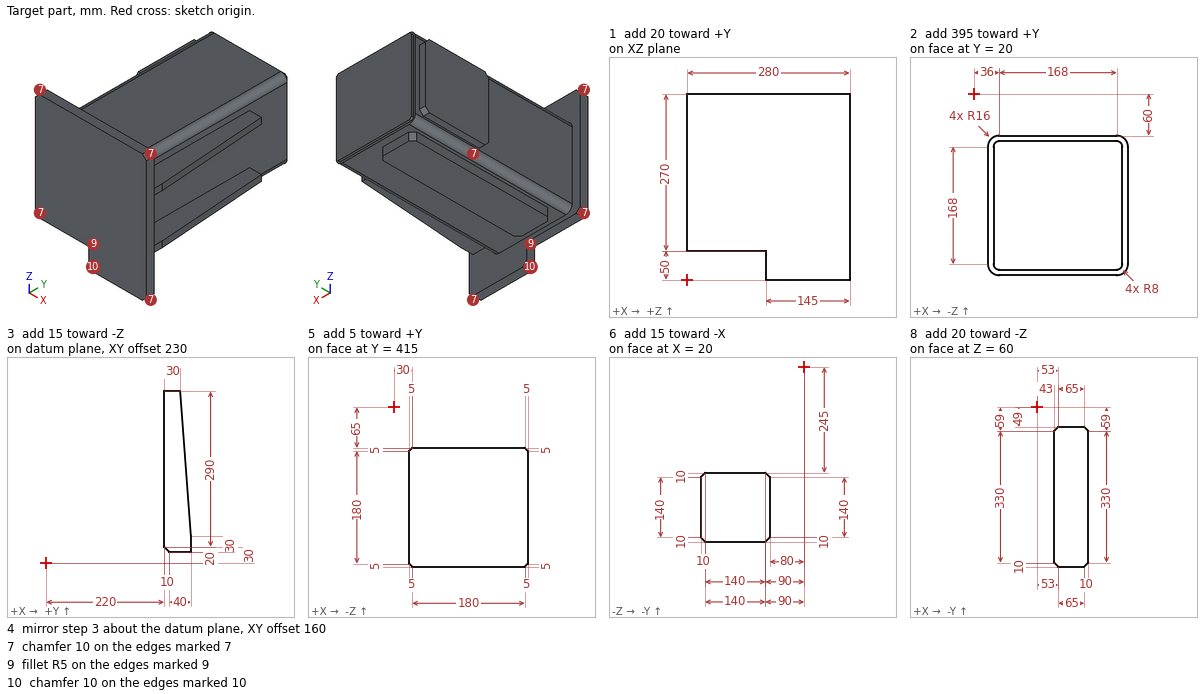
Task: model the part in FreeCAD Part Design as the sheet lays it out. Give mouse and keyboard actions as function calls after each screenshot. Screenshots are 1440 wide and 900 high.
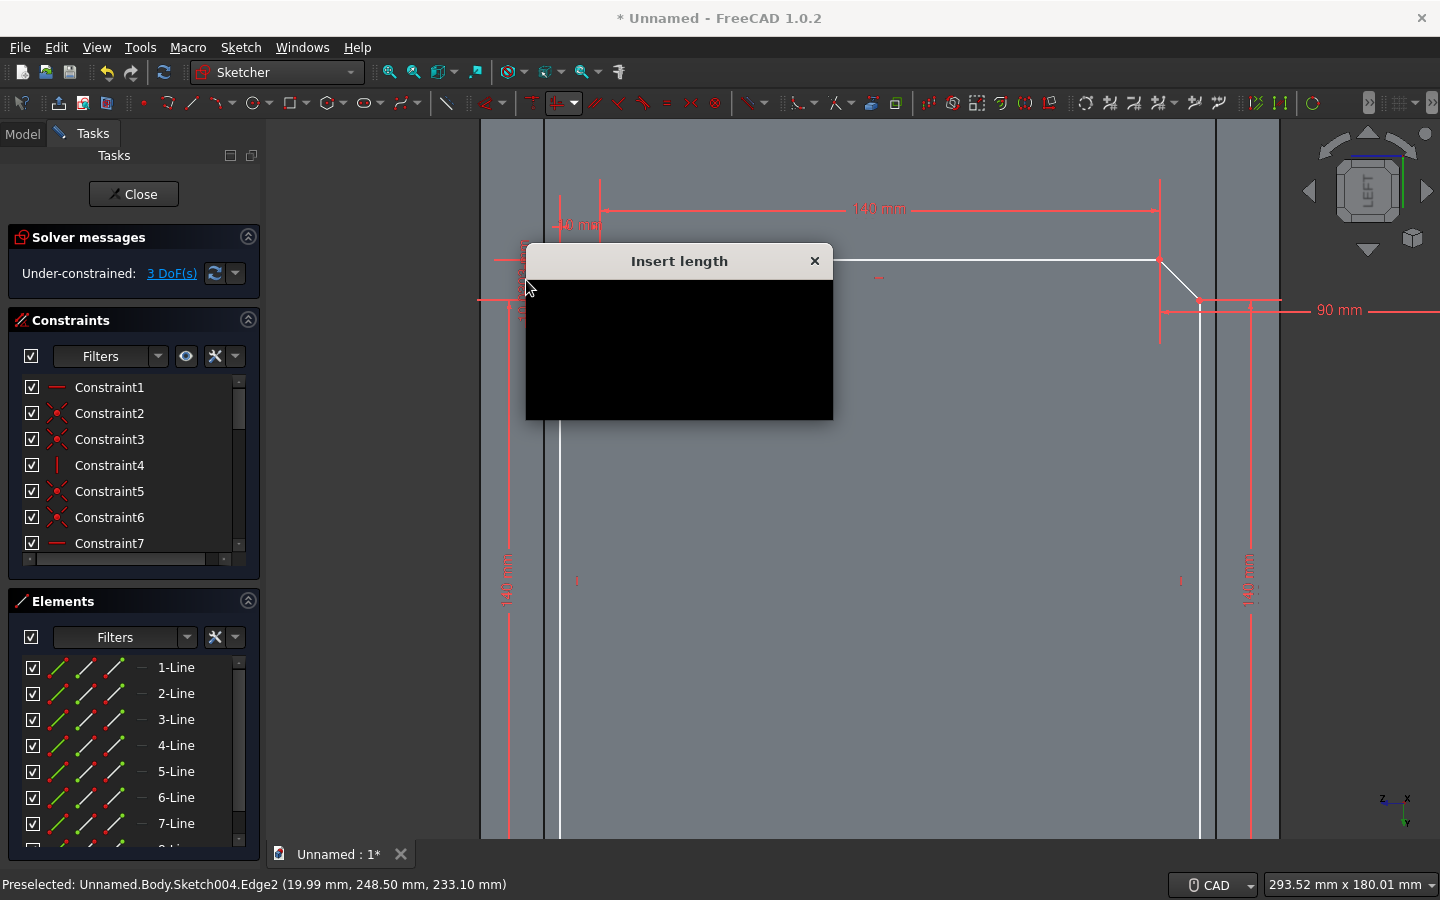
text(10)
key(Return)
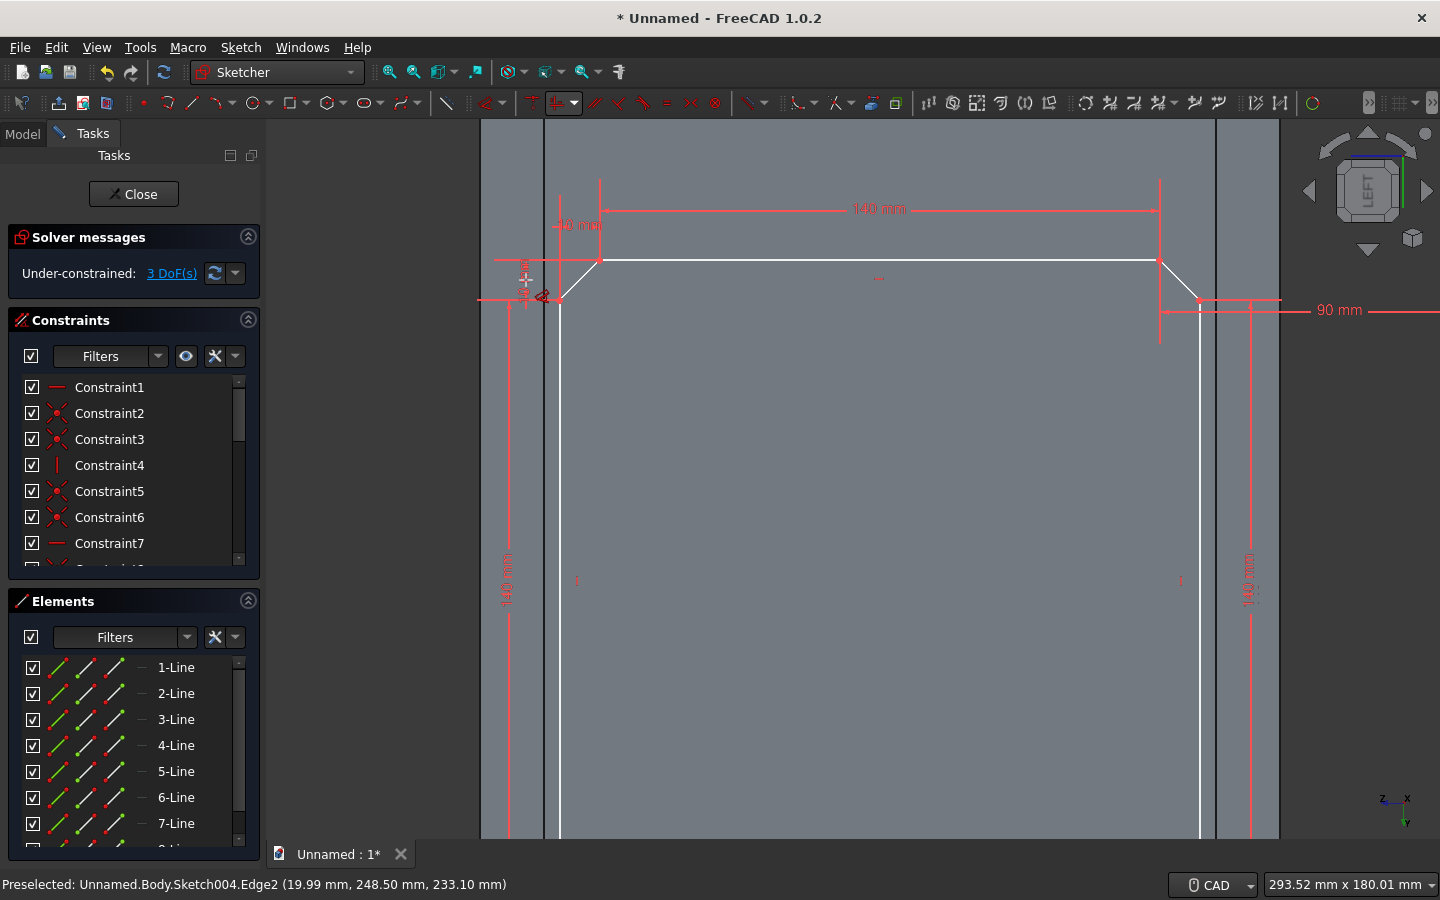
scroll(591, 277, down, 2)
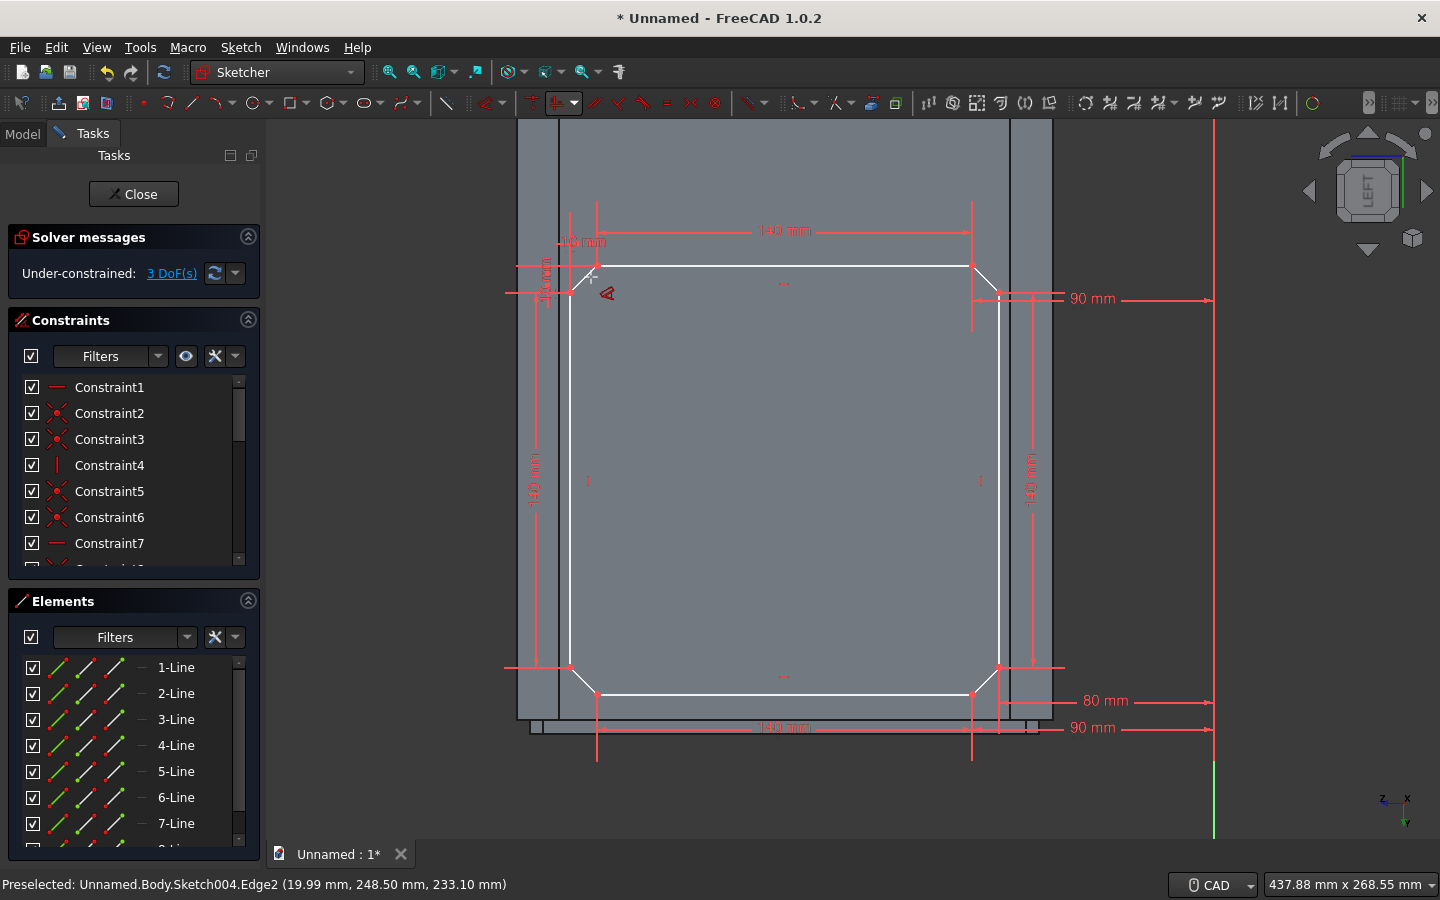
scroll(578, 676, up, 2)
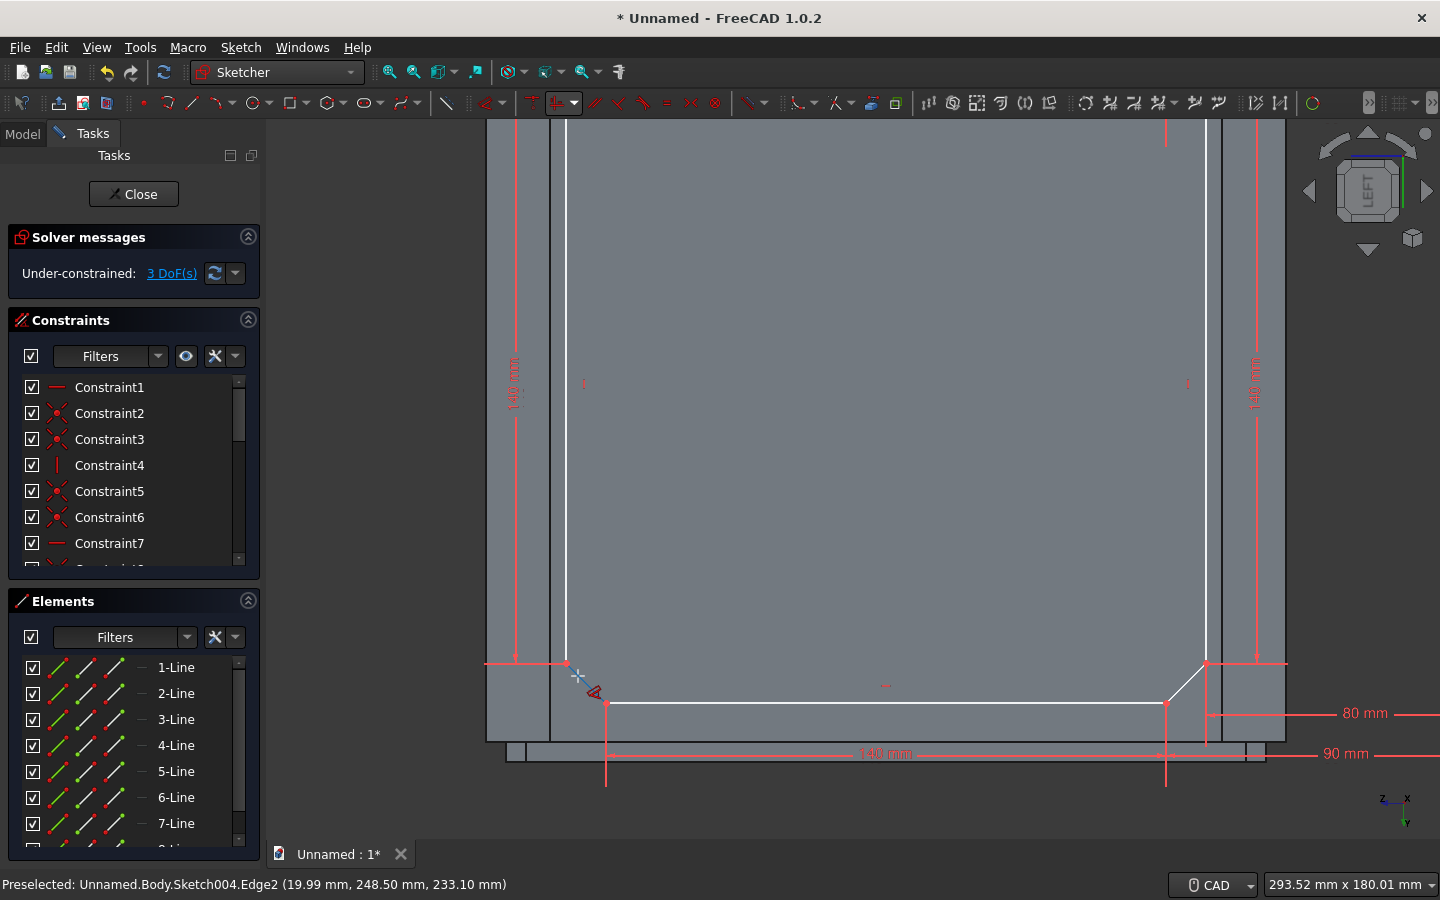
click(578, 676)
click(532, 683)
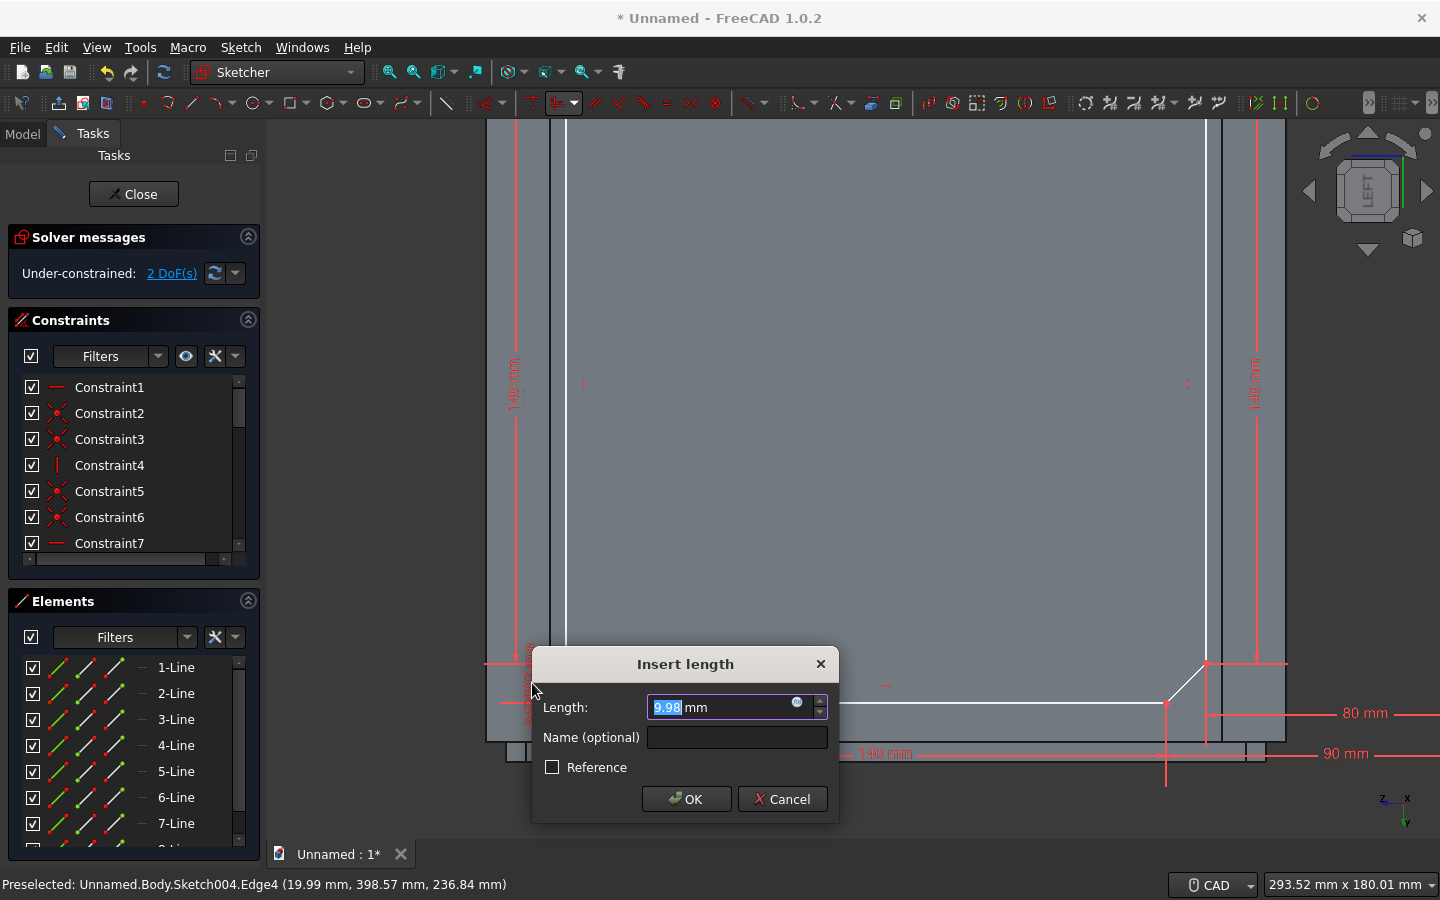
text(10)
key(Return)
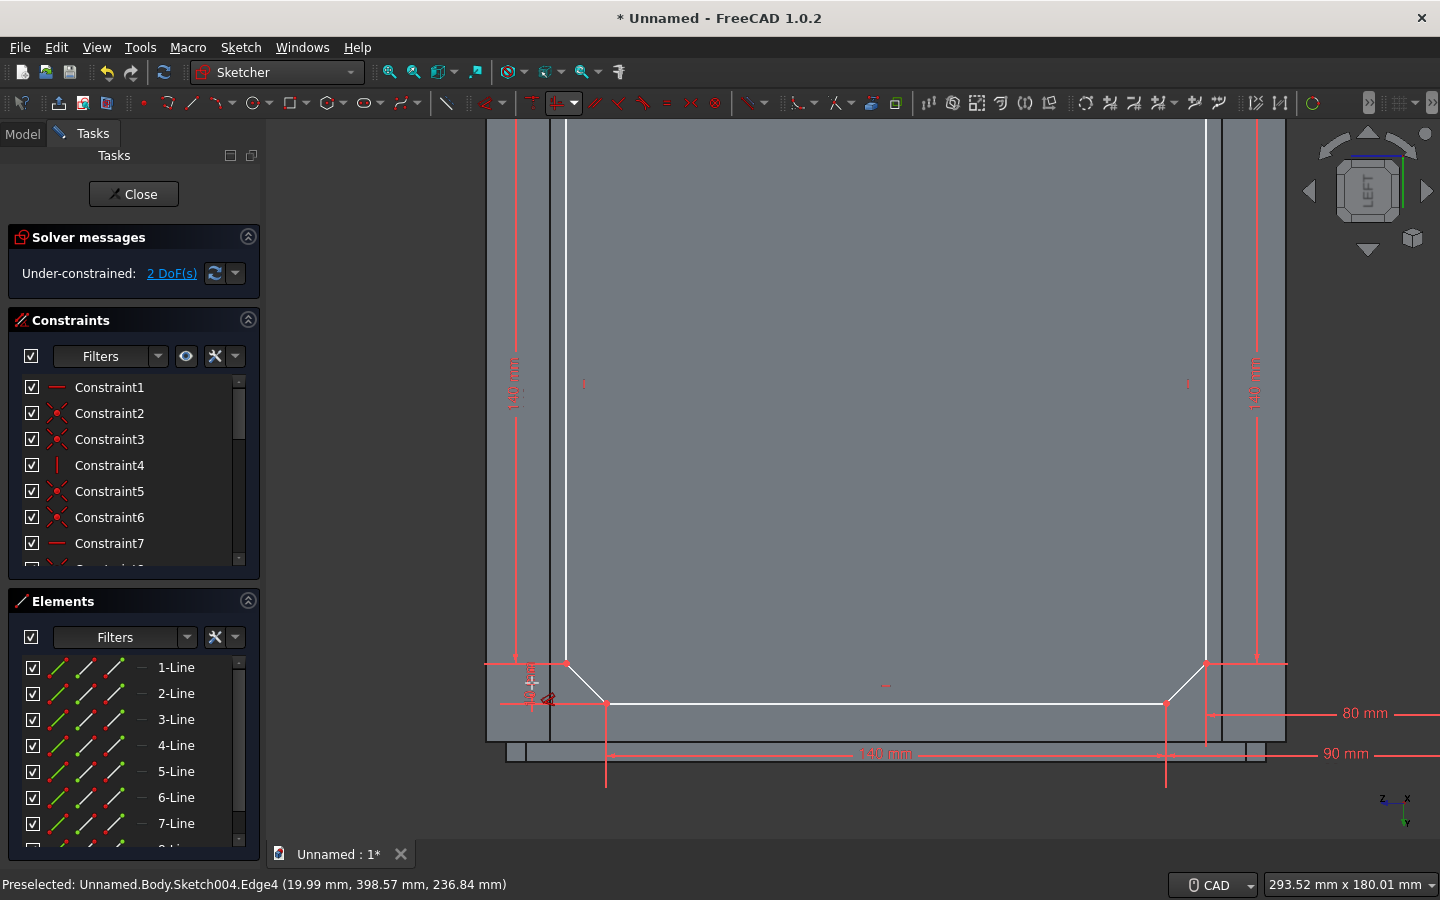
click(1178, 692)
click(1240, 684)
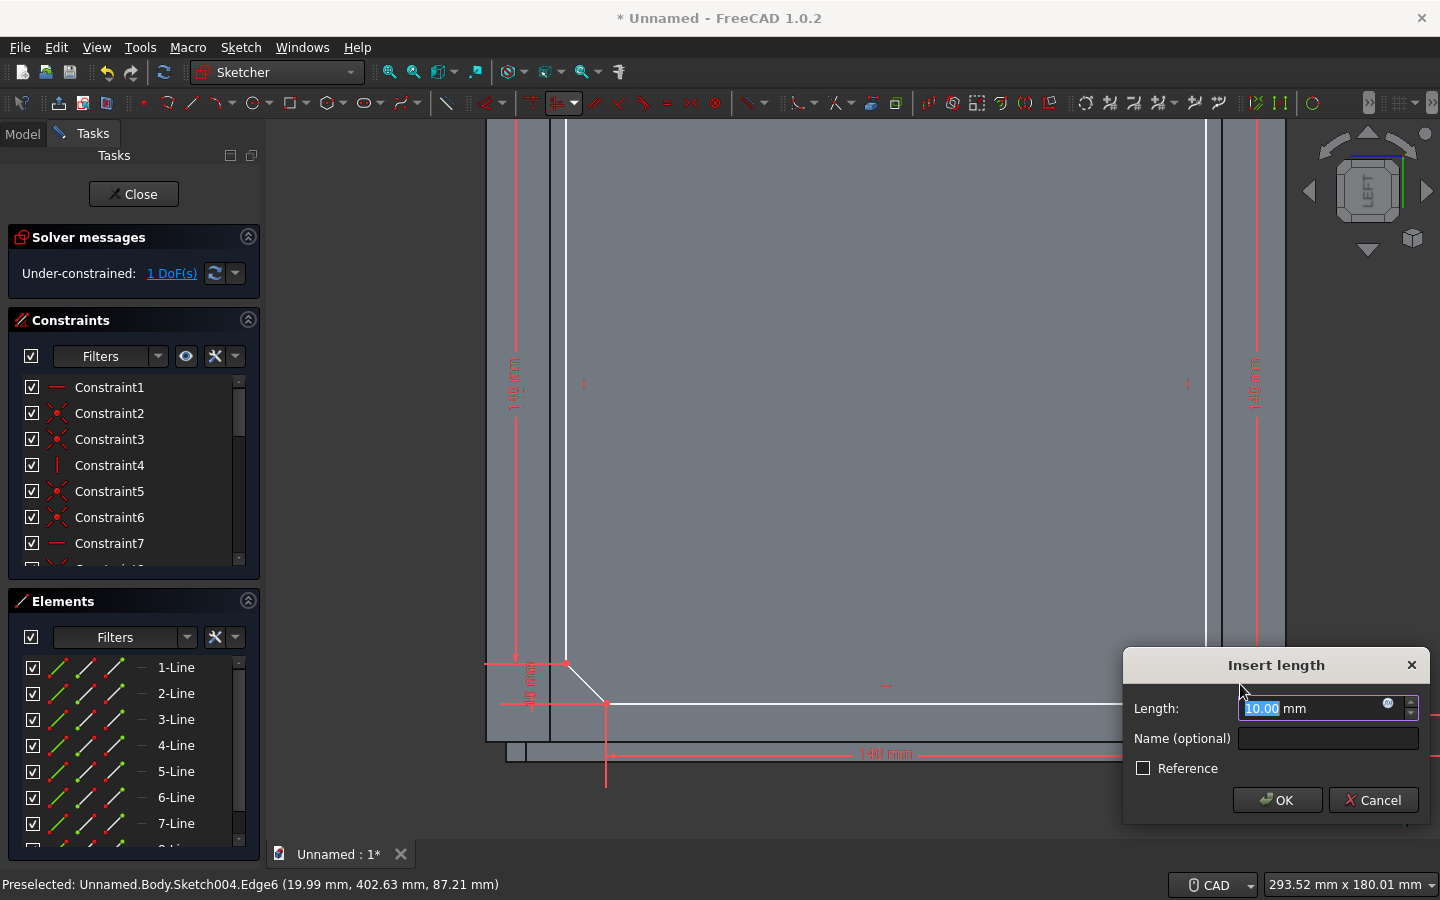
text(10)
key(Return)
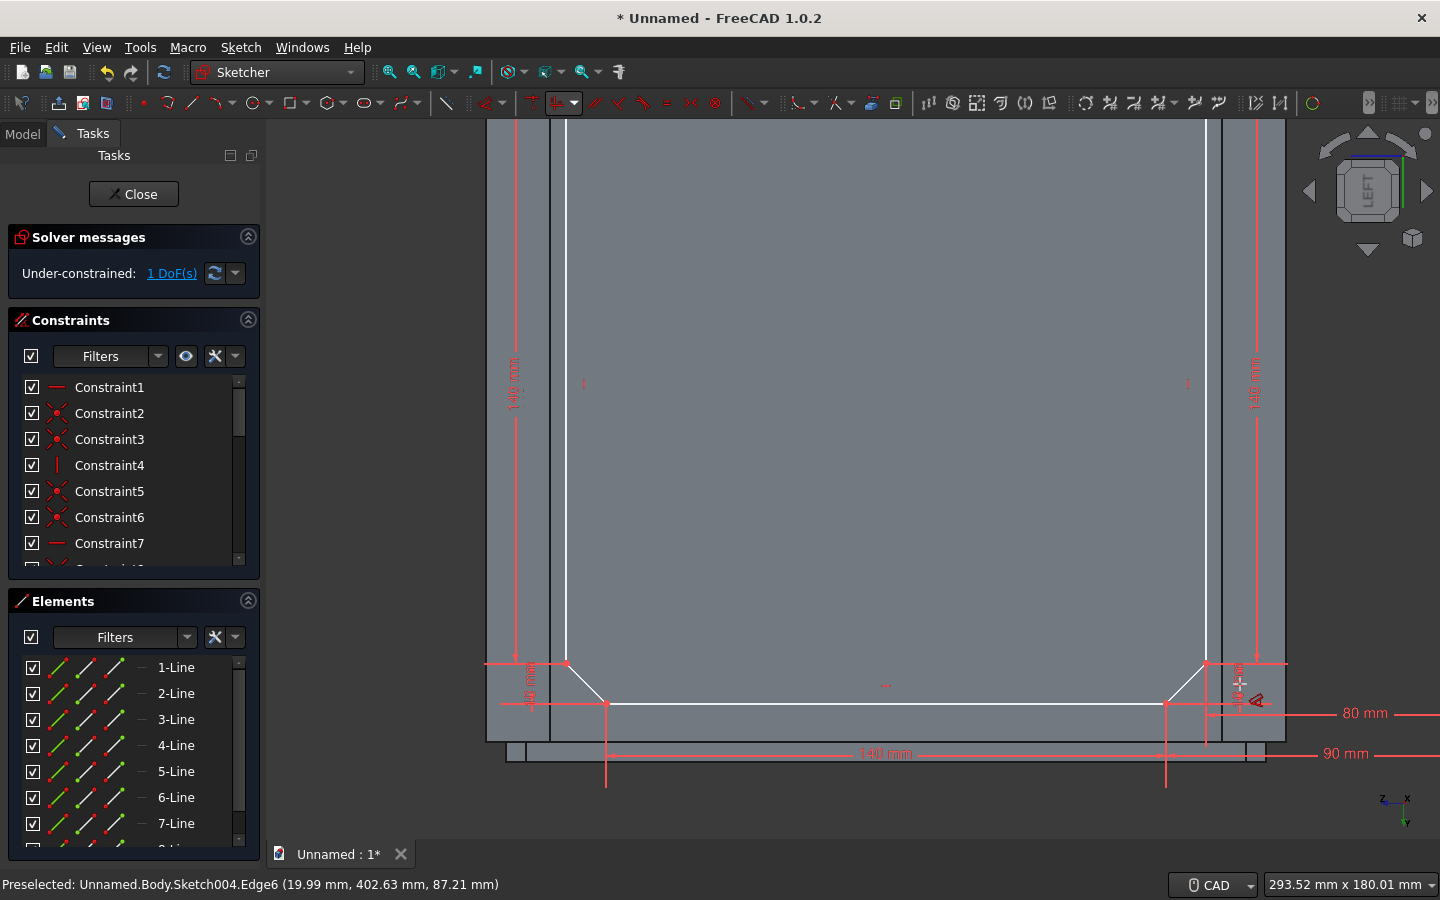
scroll(578, 676, down, 2)